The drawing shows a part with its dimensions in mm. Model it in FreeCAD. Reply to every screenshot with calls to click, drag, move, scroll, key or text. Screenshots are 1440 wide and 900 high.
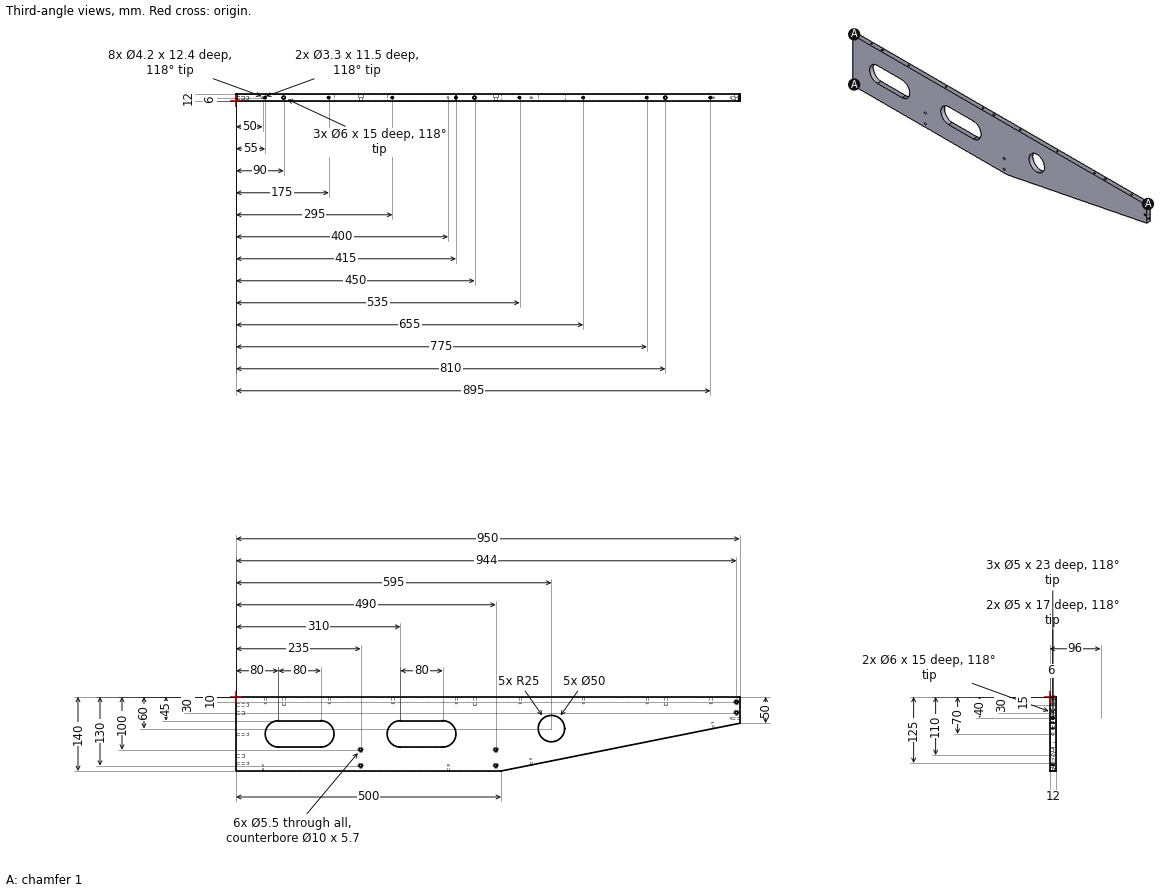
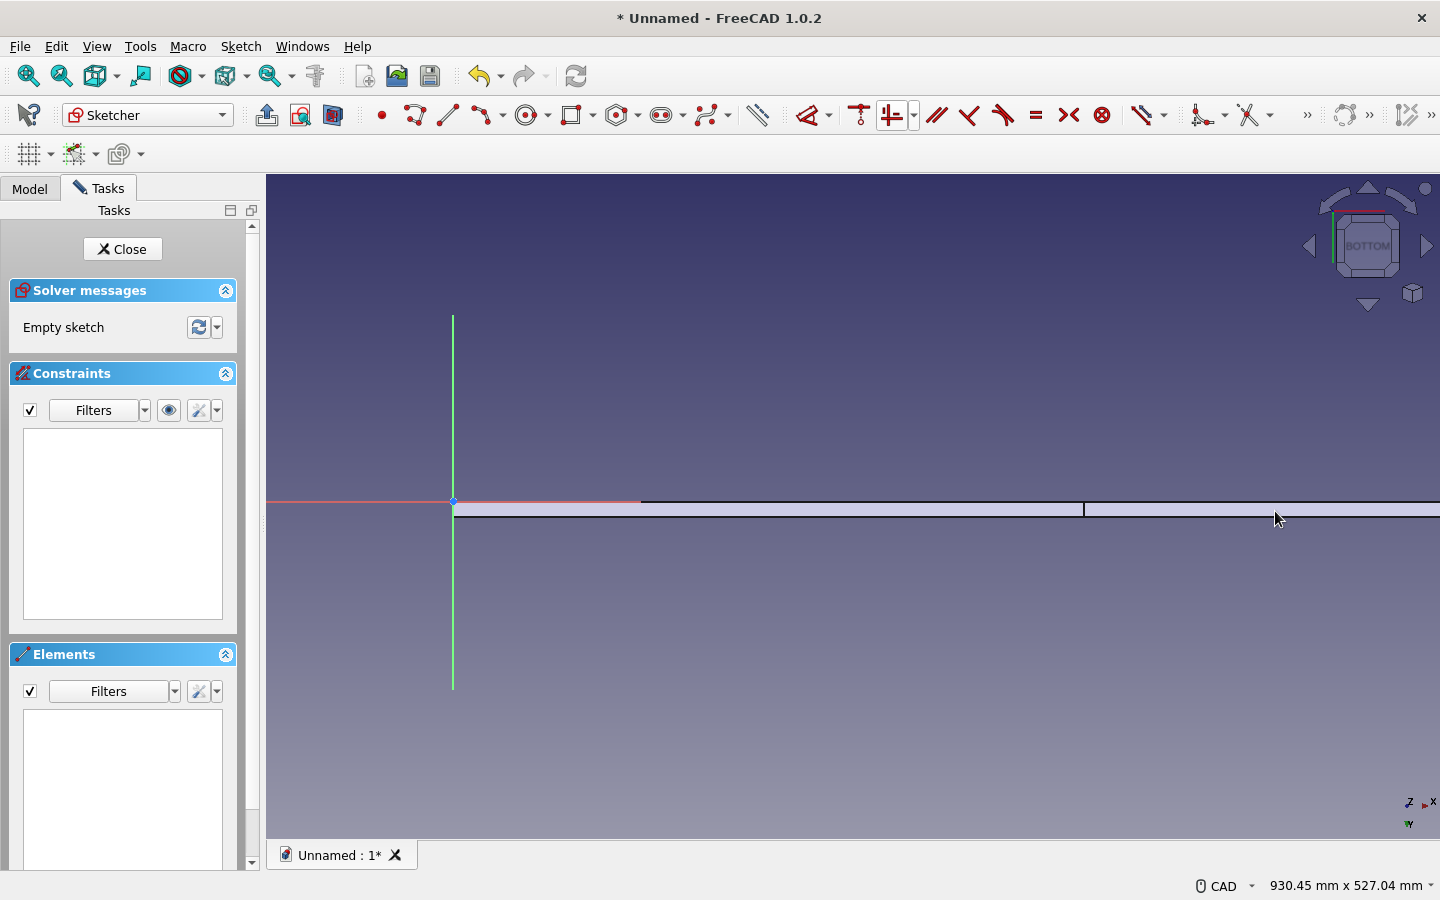
scroll(549, 507, up, 2)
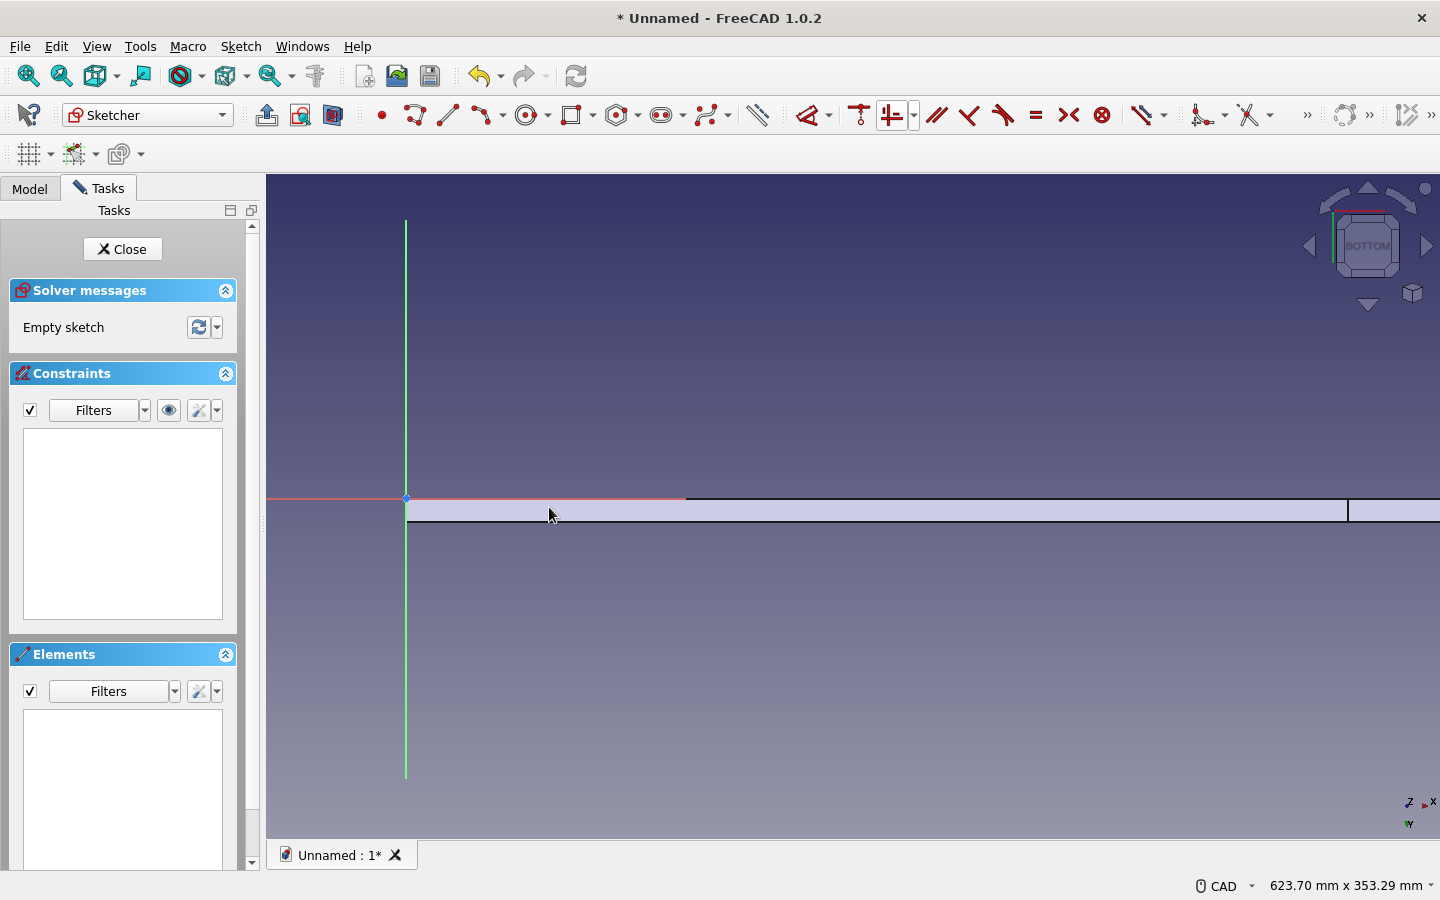
click(526, 116)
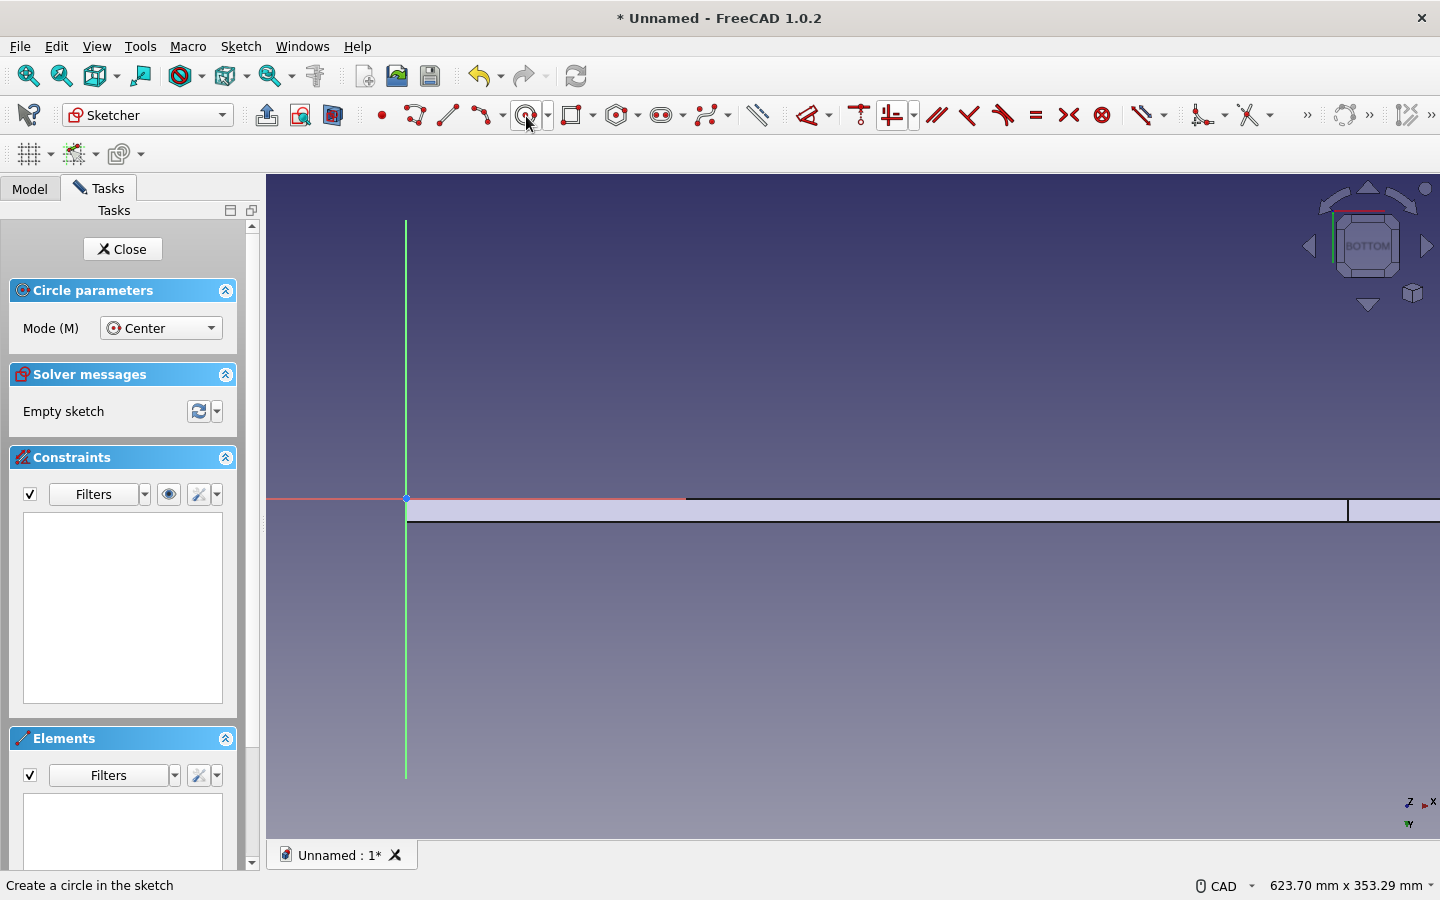
scroll(501, 510, up, 10)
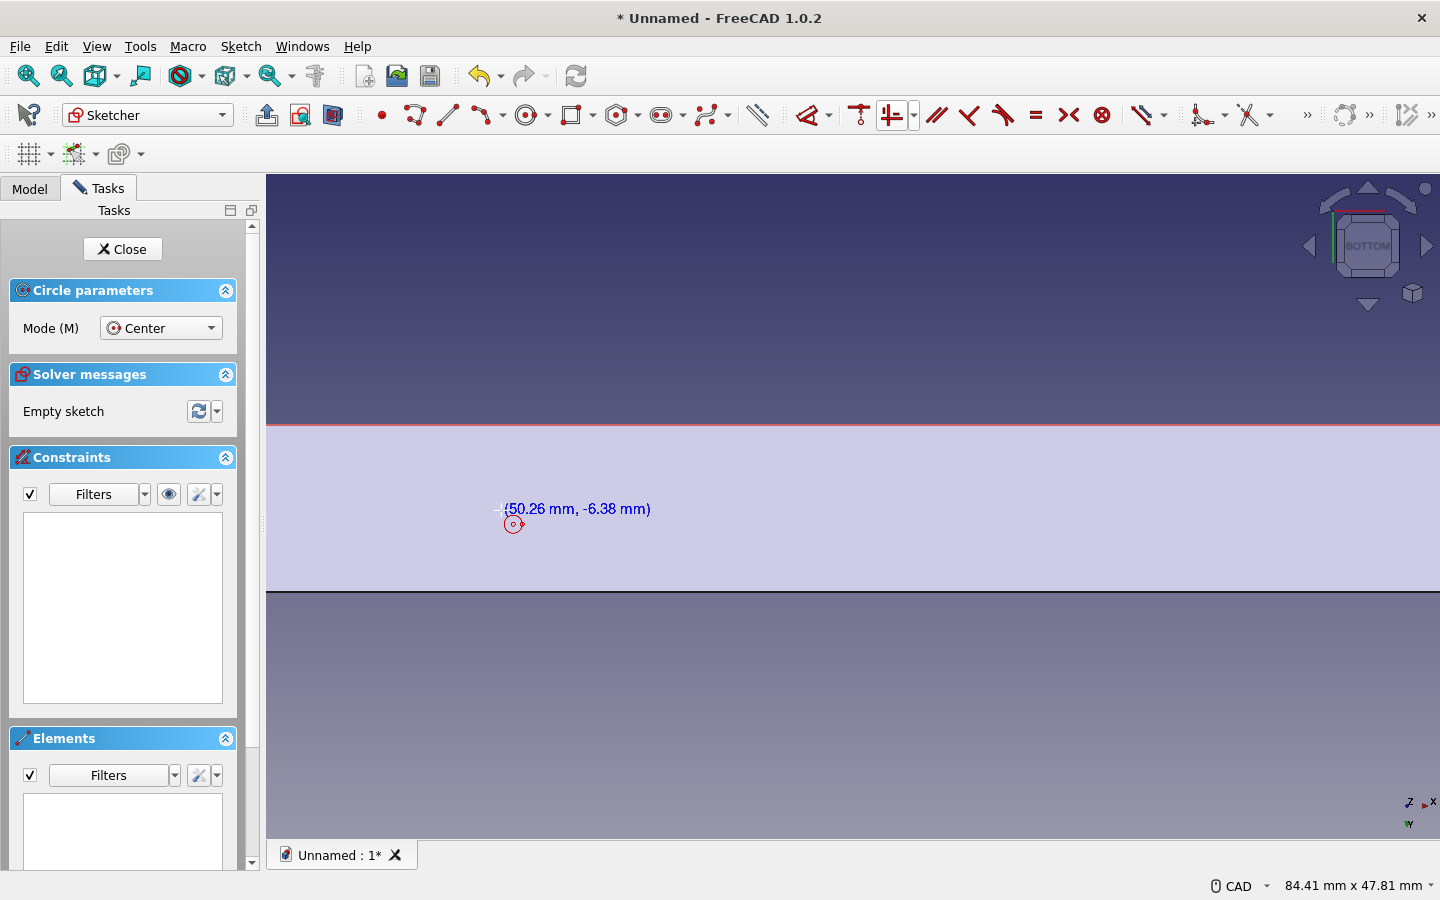
scroll(501, 511, down, 10)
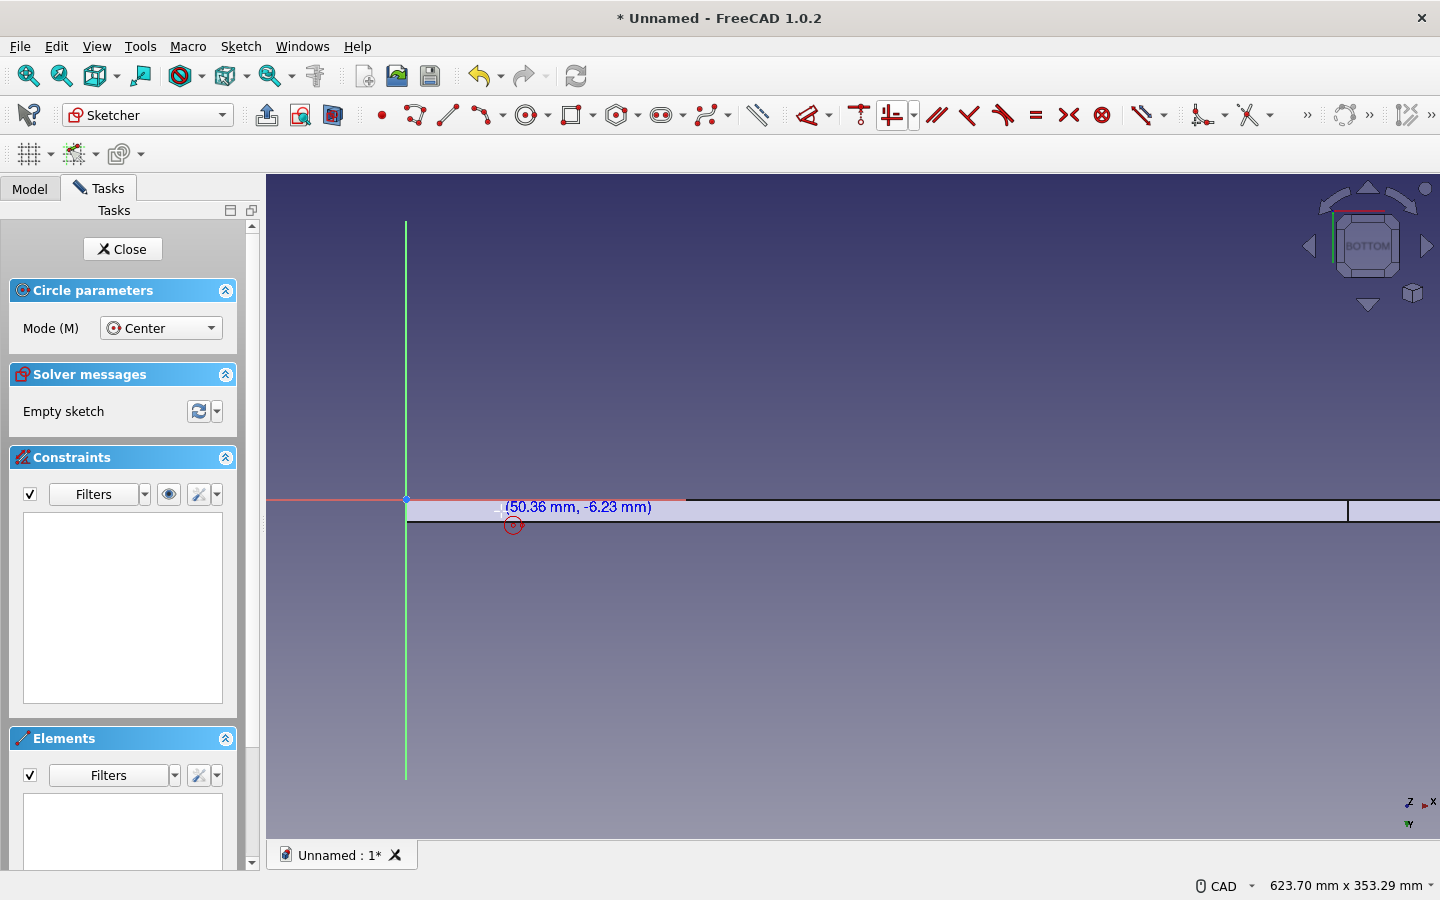
scroll(501, 511, up, 2)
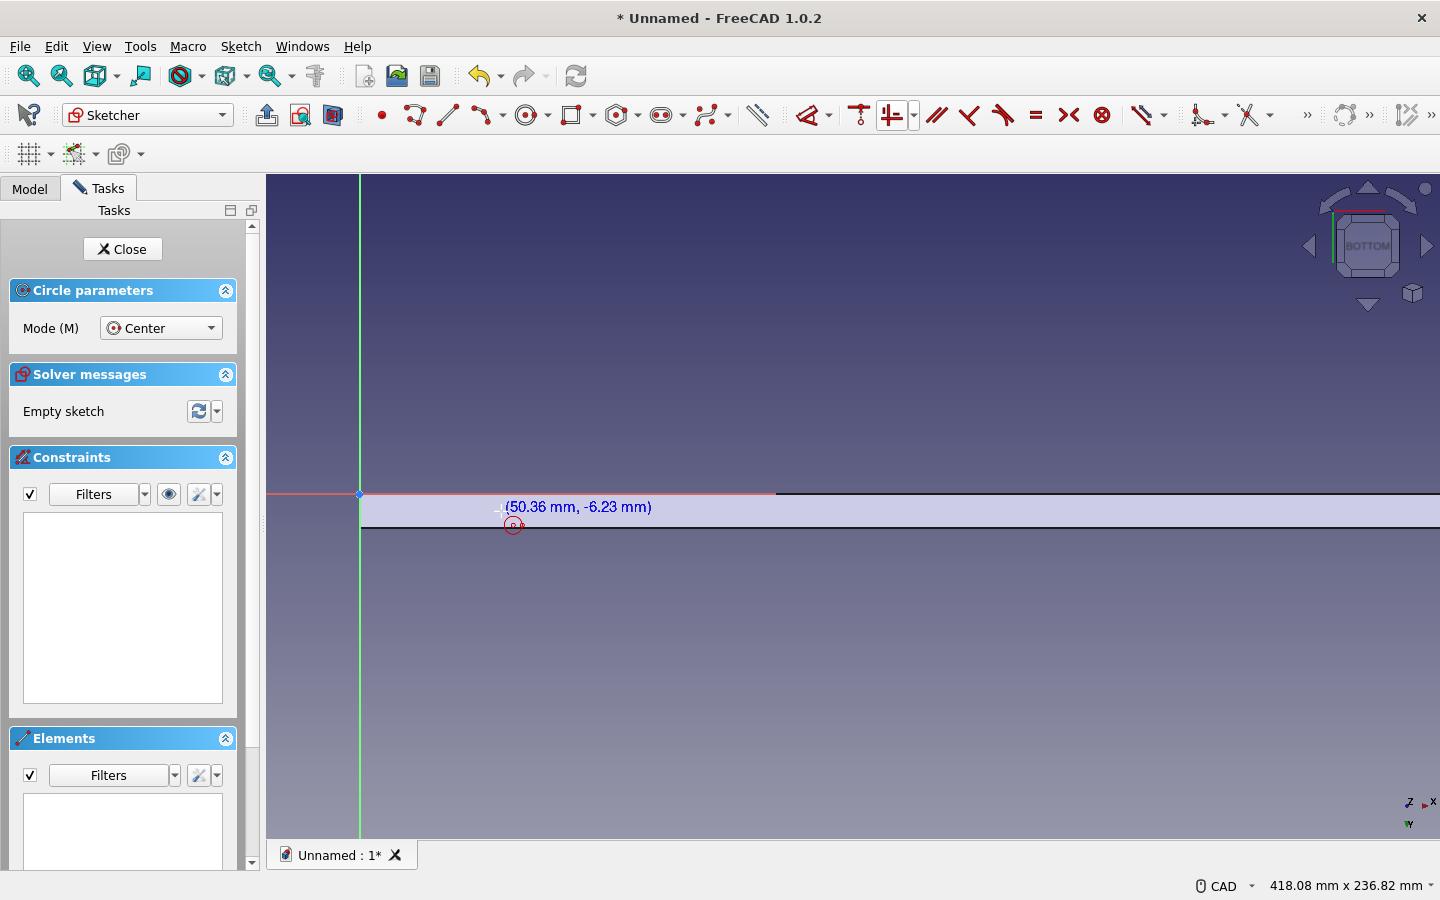
click(500, 511)
move(503, 514)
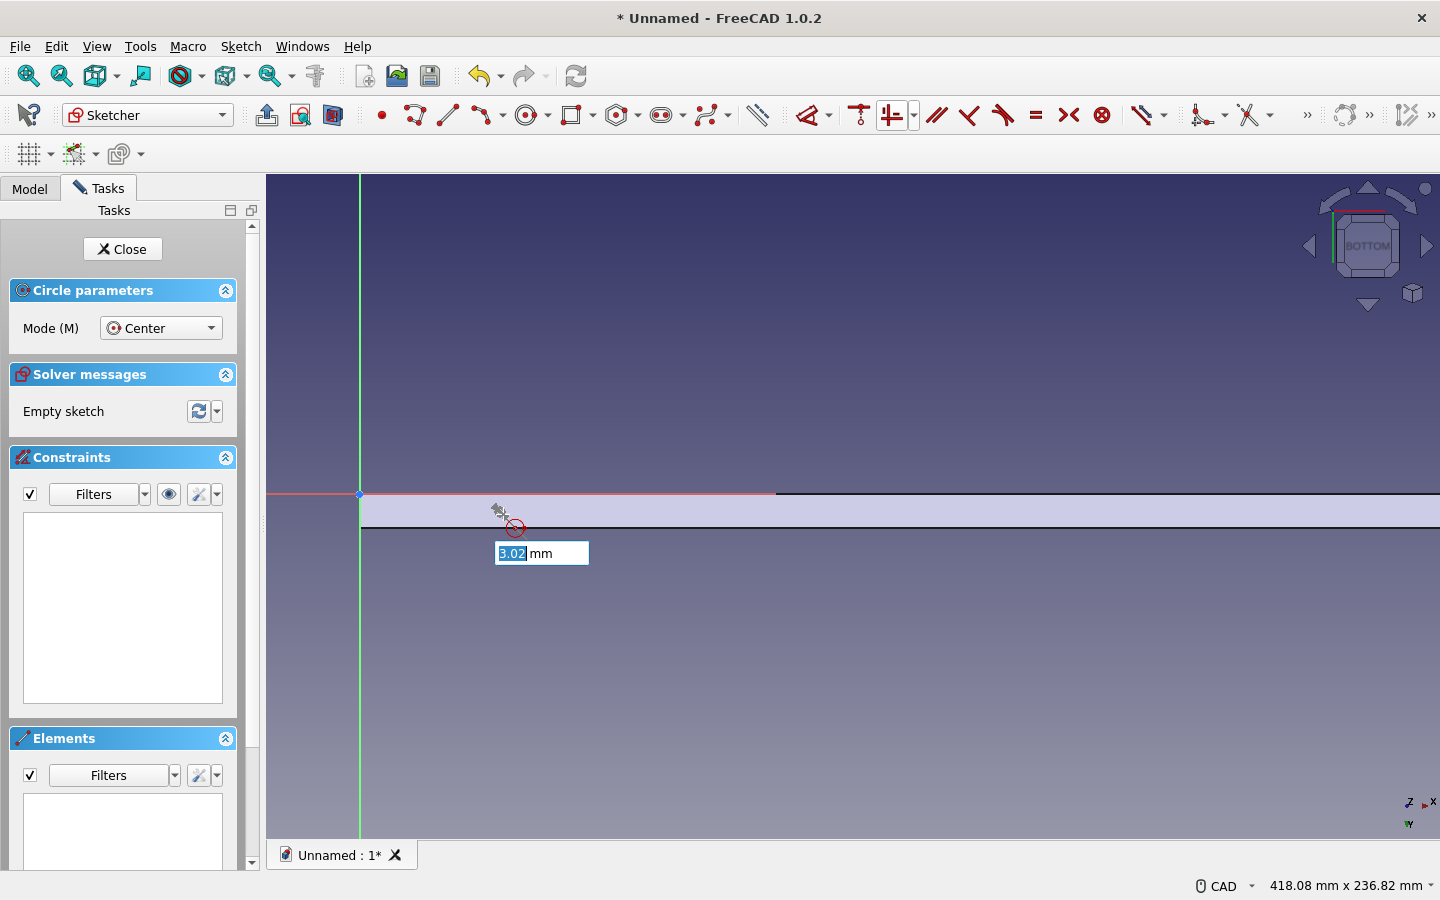
text(3.3)
key(Return)